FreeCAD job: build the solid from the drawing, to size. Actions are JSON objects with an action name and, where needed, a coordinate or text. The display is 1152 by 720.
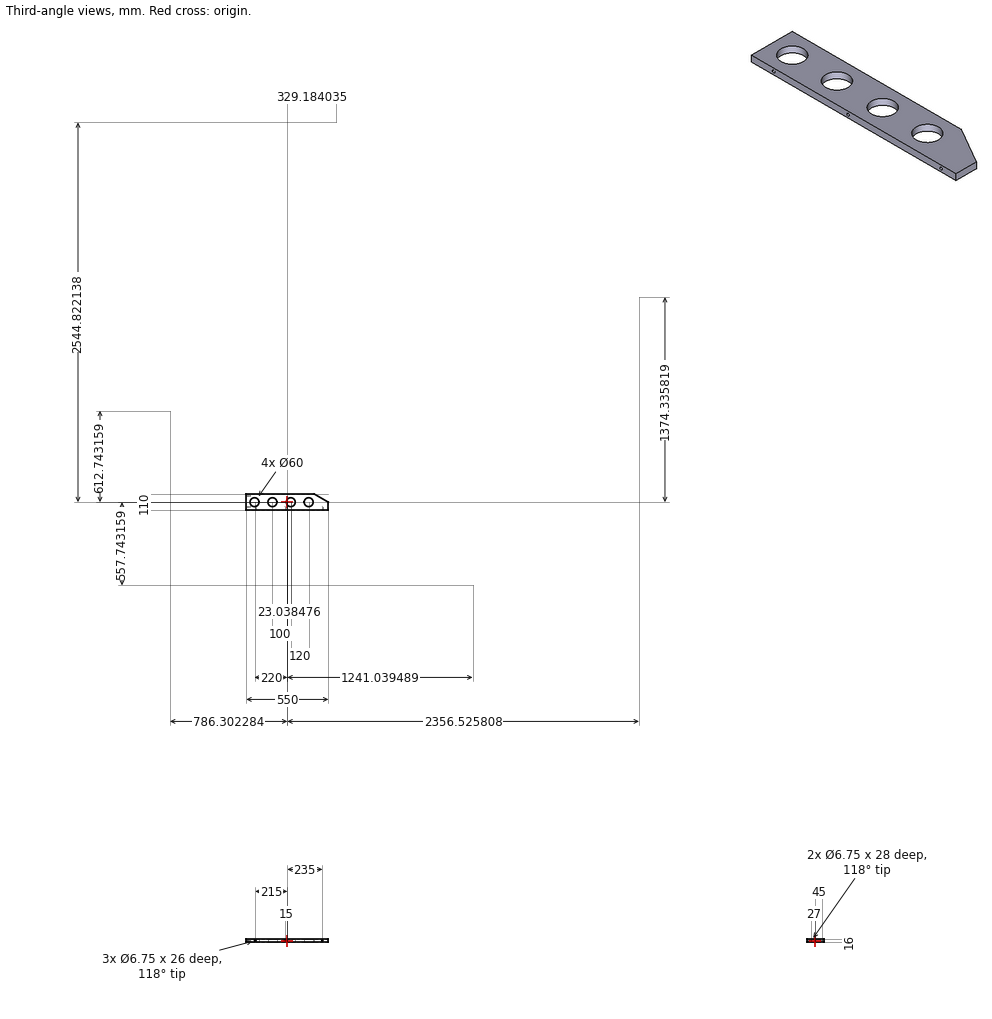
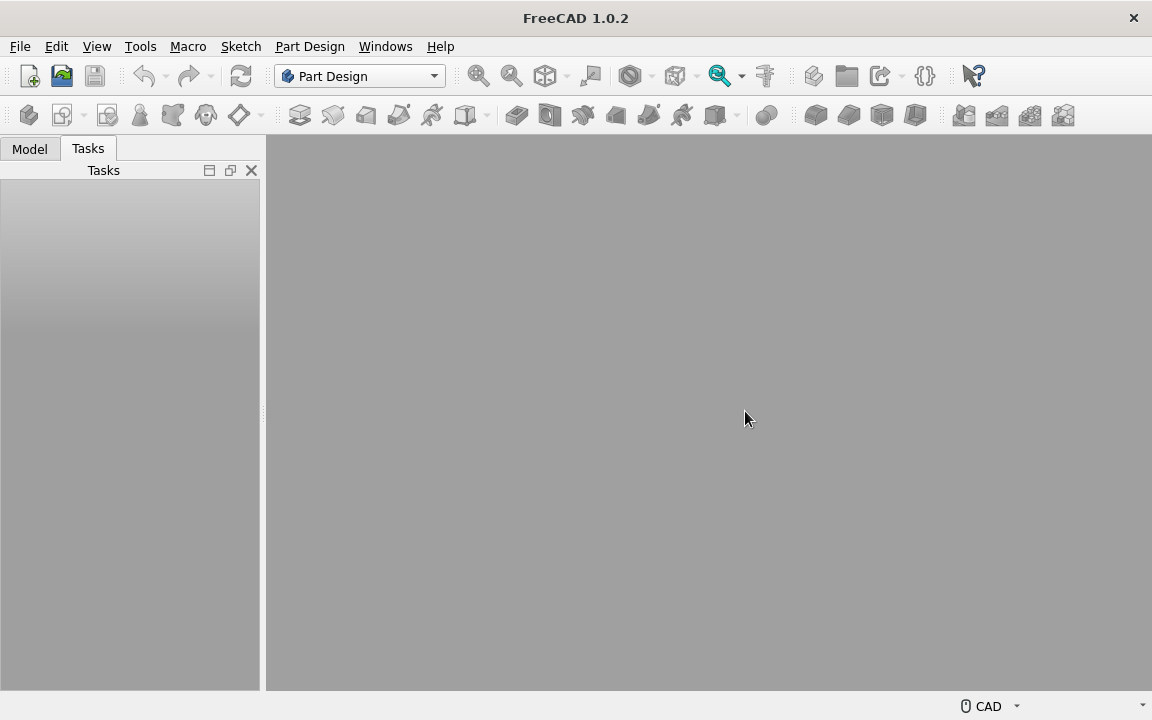
{"action": "key", "text": "ctrl+n"}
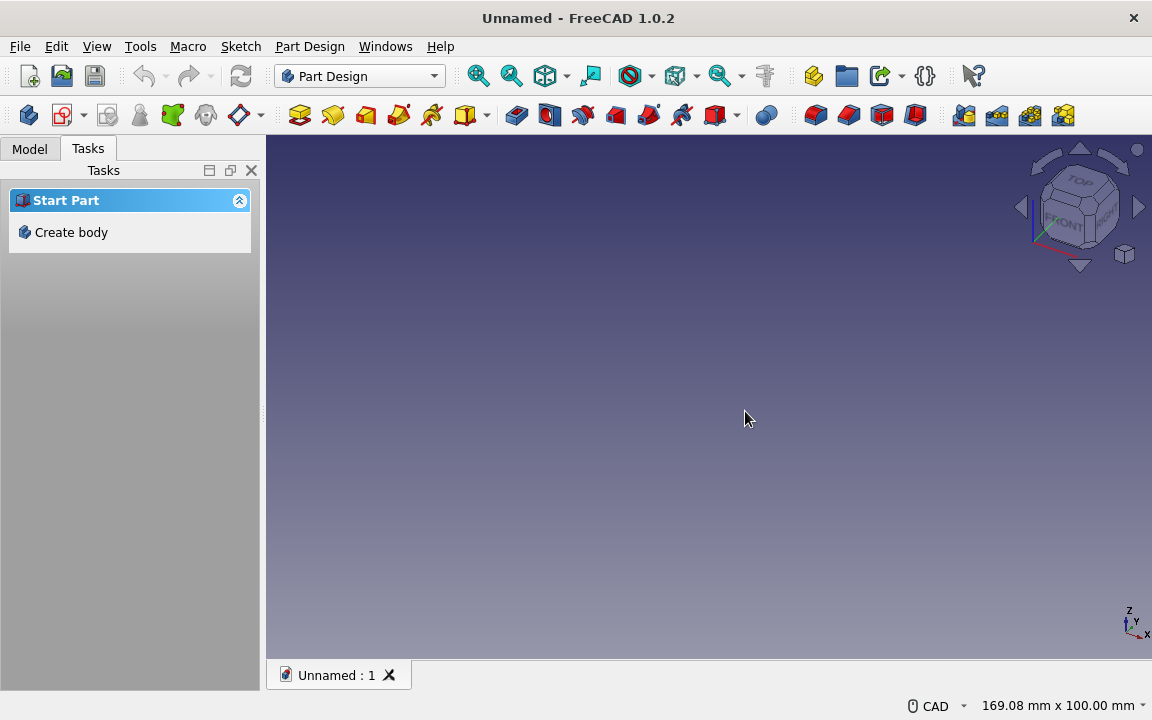
{"action": "left_click", "coordinate": [62, 116]}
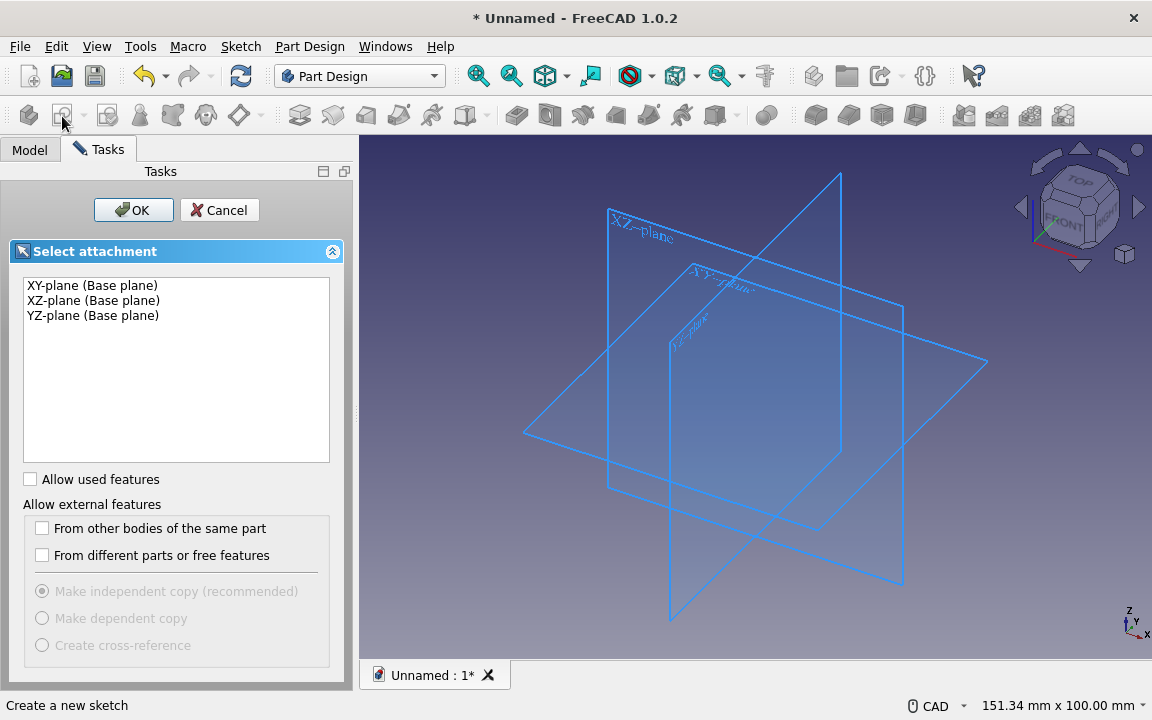
{"action": "left_click", "coordinate": [84, 286]}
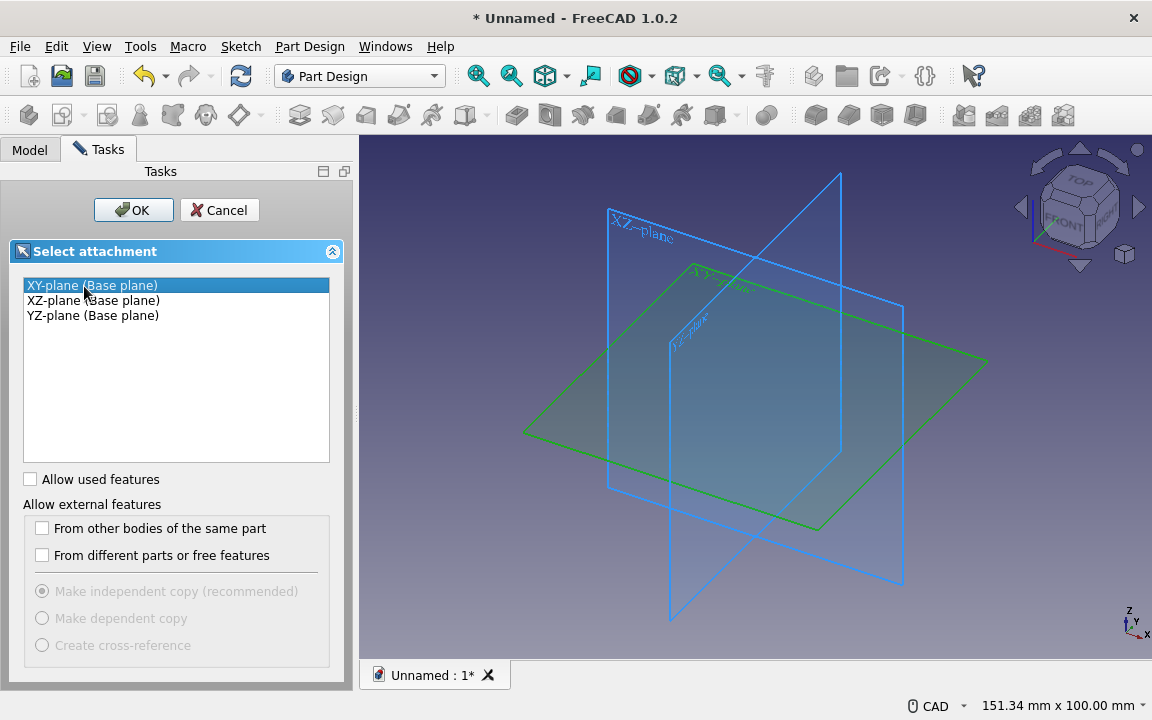
{"action": "left_click", "coordinate": [134, 210]}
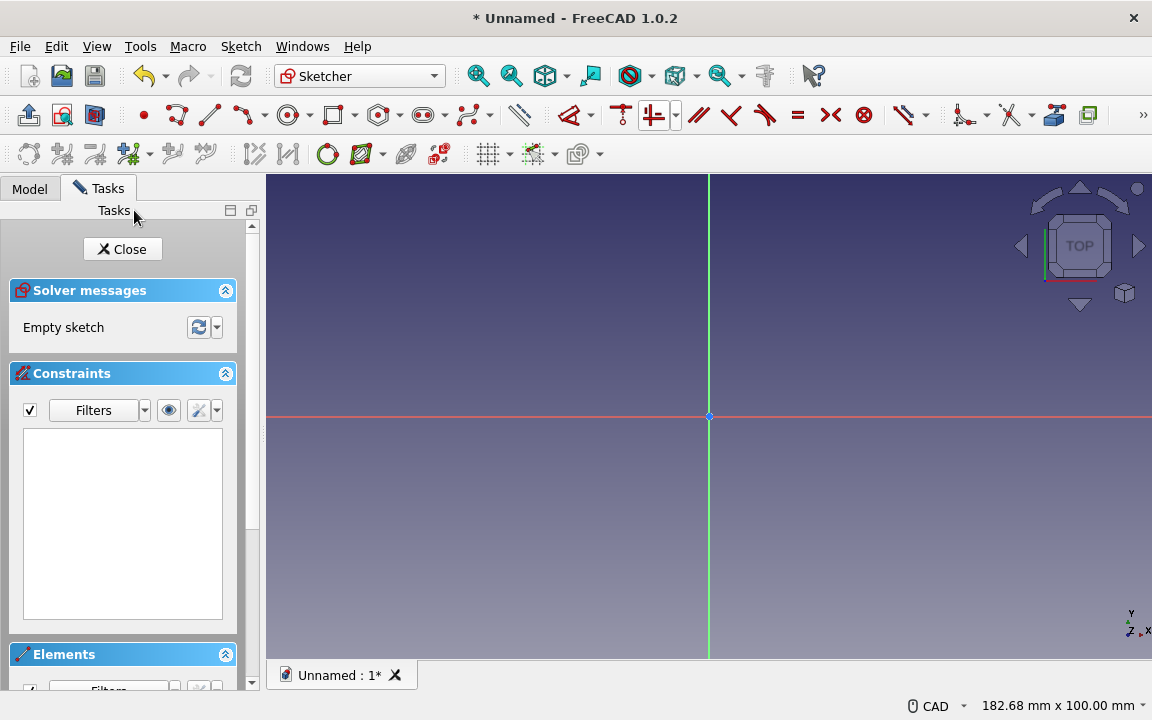
{"action": "scroll", "coordinate": [623, 416], "scroll_direction": "down", "scroll_amount": 8}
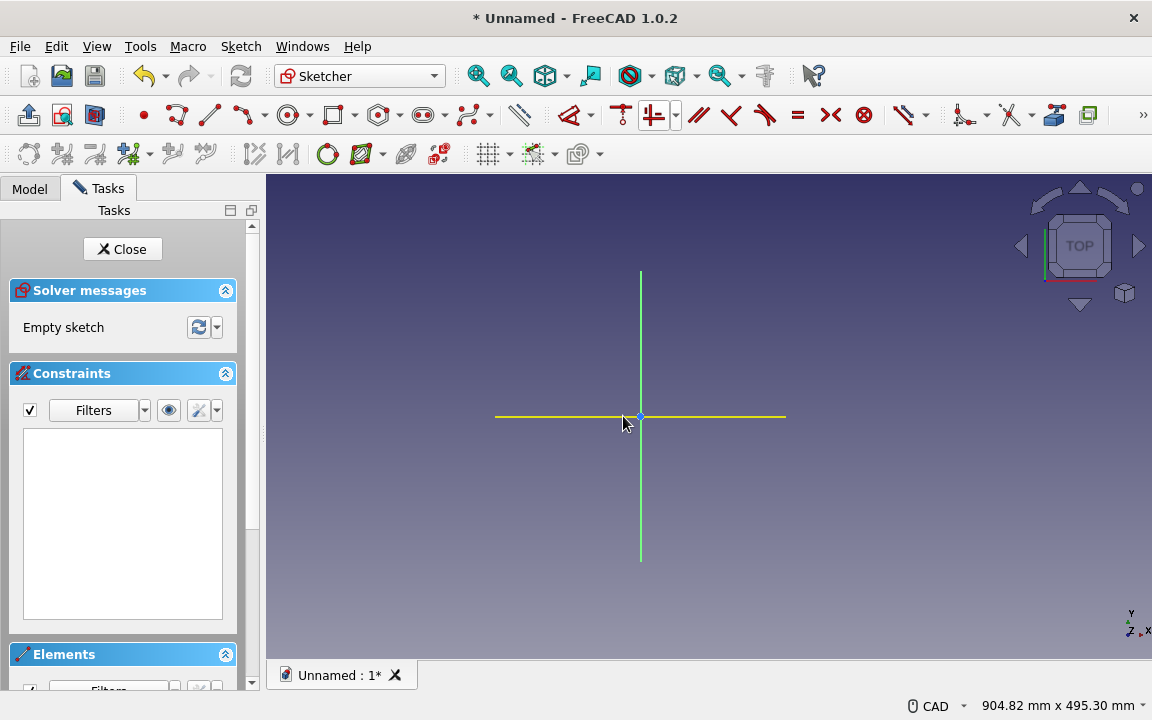
{"action": "key", "text": "g v"}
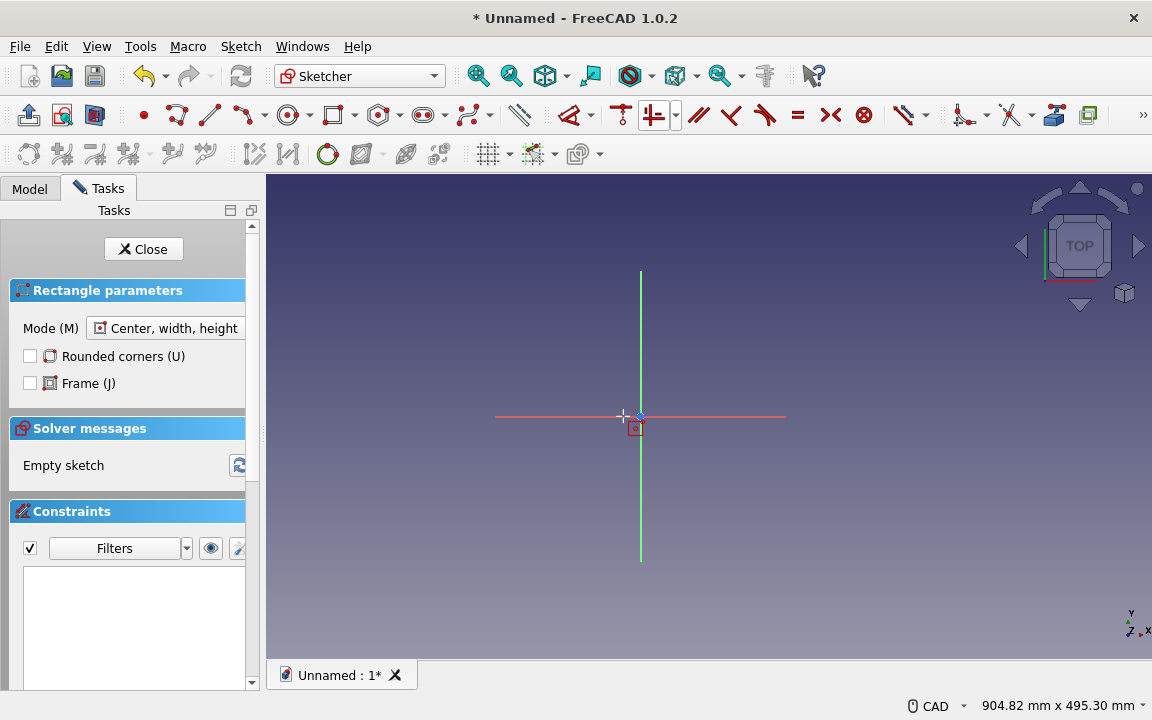
{"action": "left_click", "coordinate": [641, 416]}
{"action": "mouse_move", "coordinate": [910, 363]}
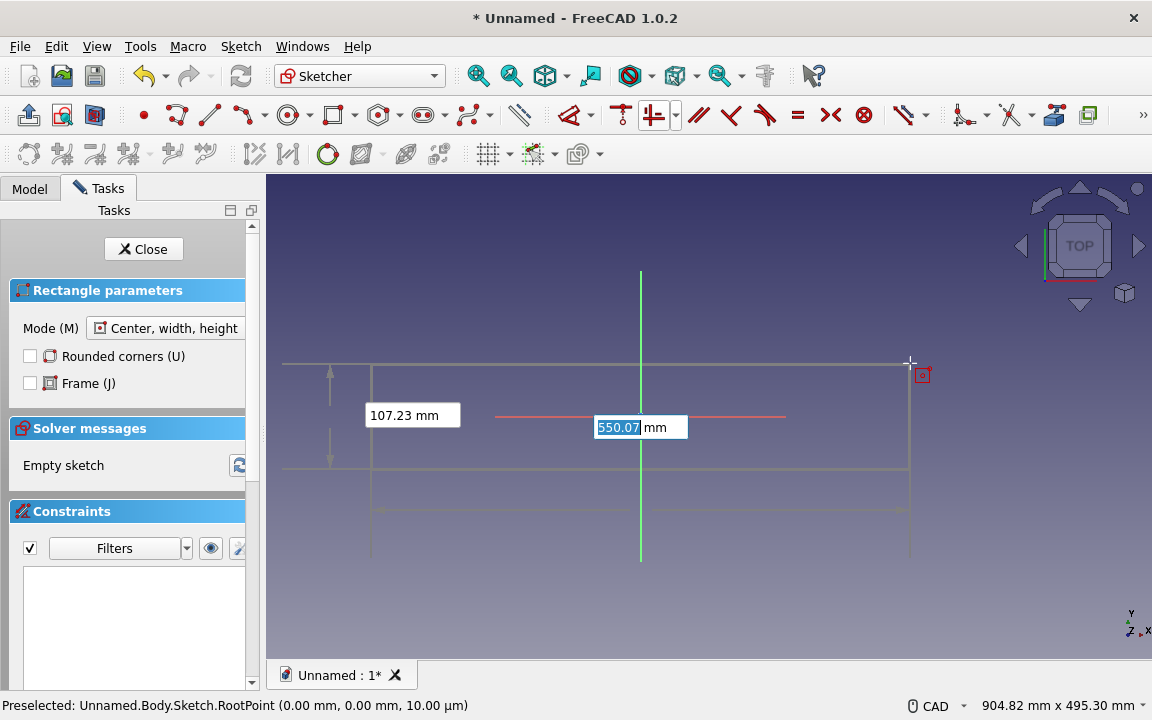
{"action": "type", "text": "550"}
{"action": "key", "text": "Tab"}
{"action": "type", "text": "110"}
{"action": "key", "text": "Return"}
{"action": "key", "text": "Escape"}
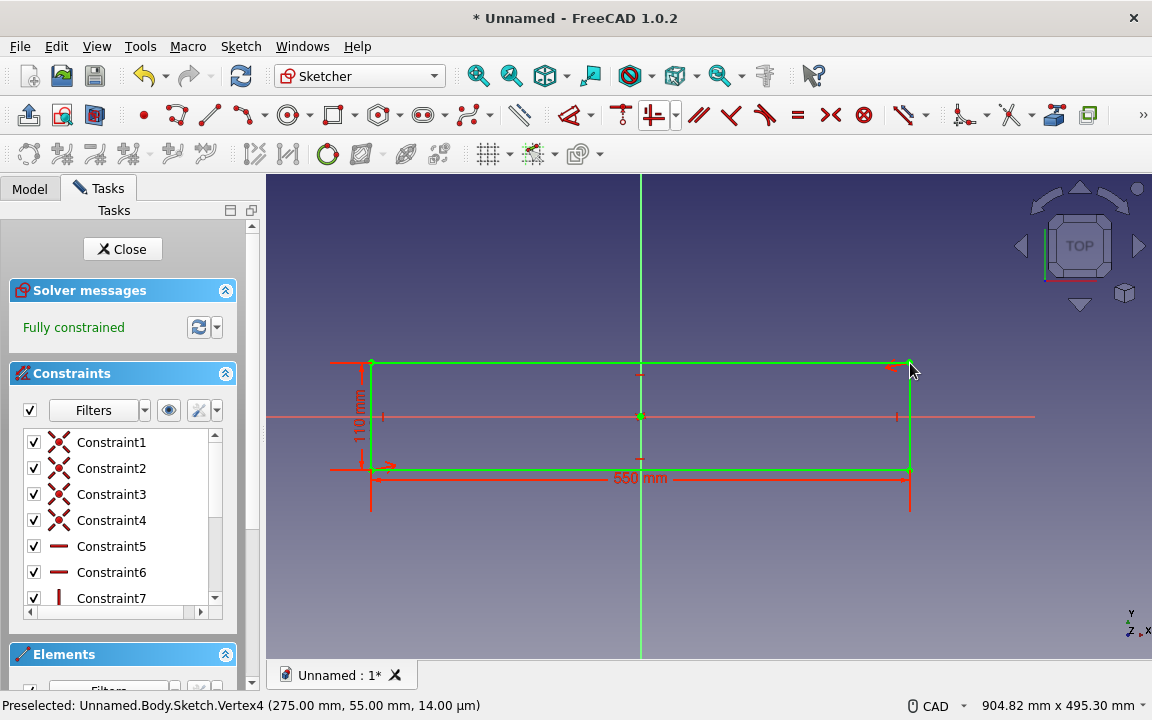
{"action": "left_click", "coordinate": [123, 249]}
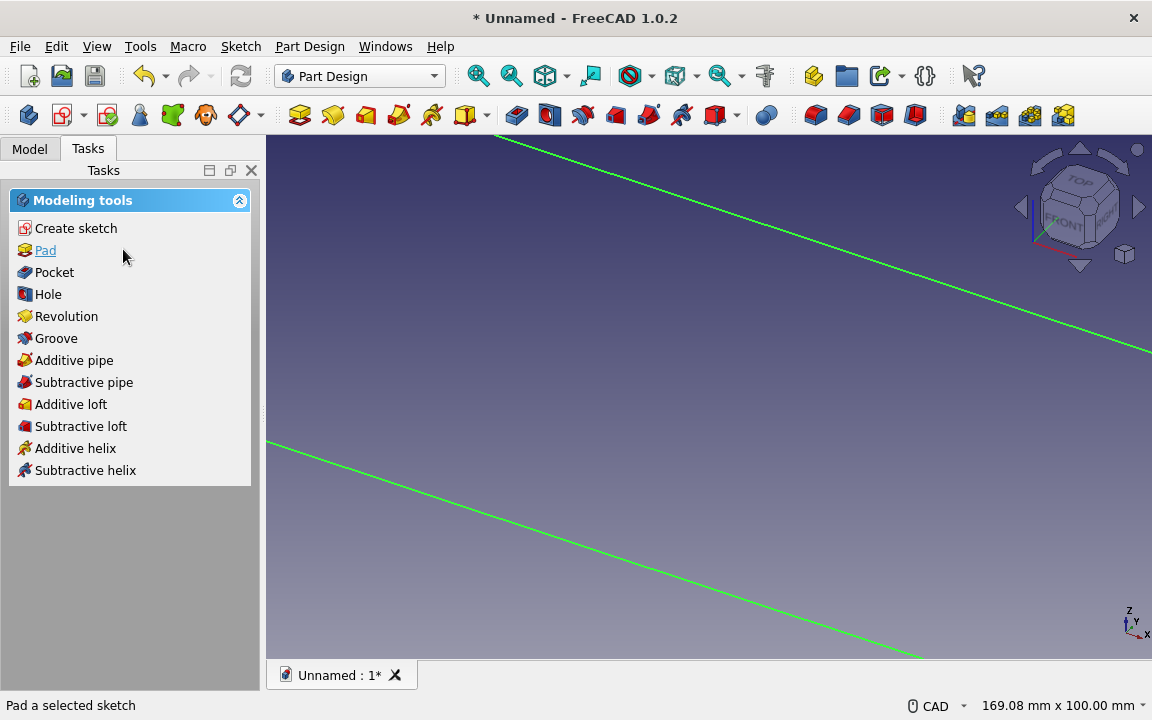
{"action": "left_click", "coordinate": [300, 116]}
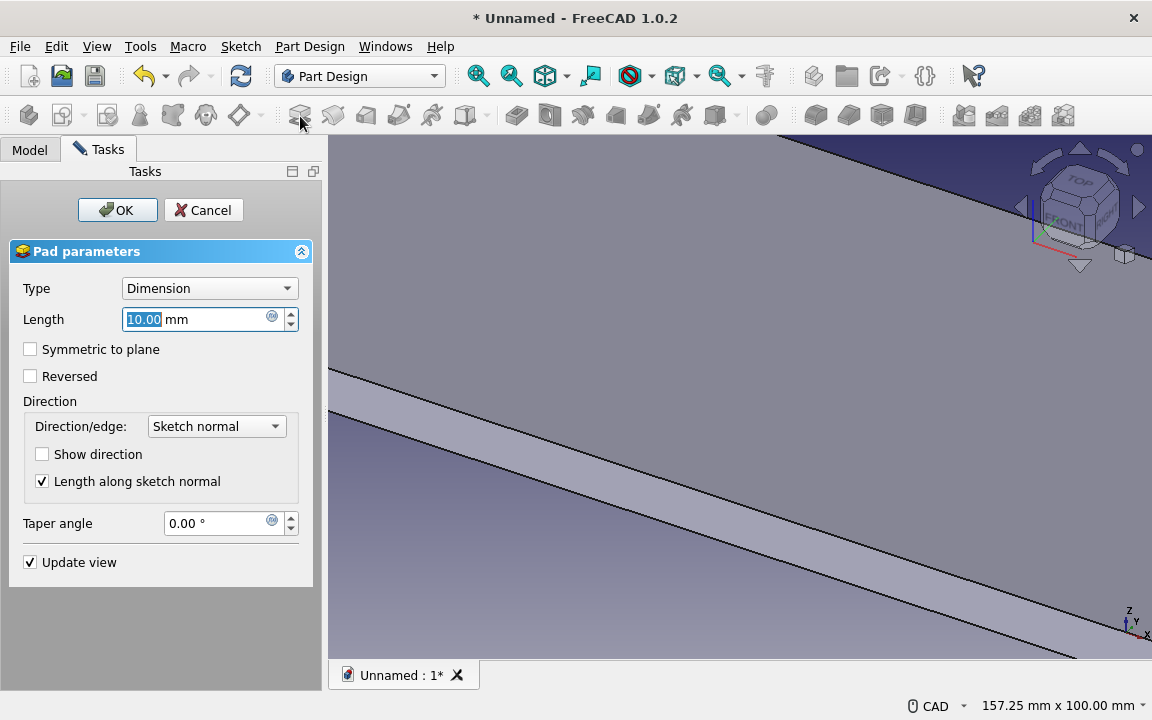
{"action": "type", "text": "16"}
{"action": "key", "text": "Tab"}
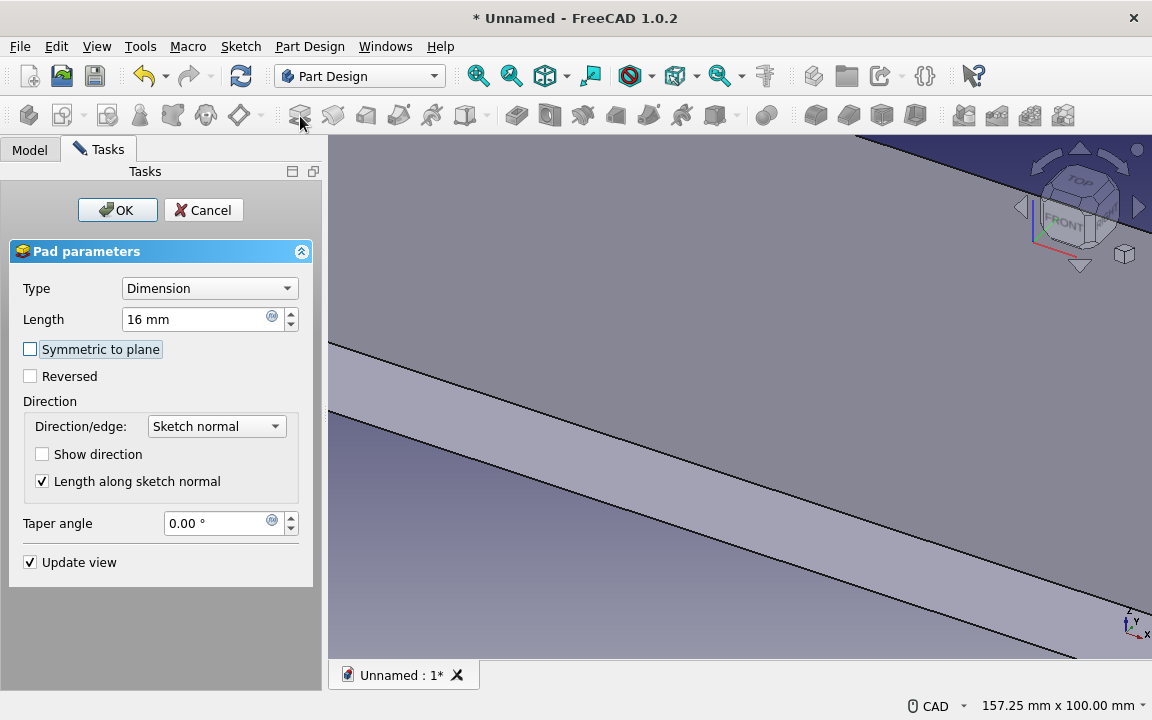
{"action": "left_click", "coordinate": [31, 349]}